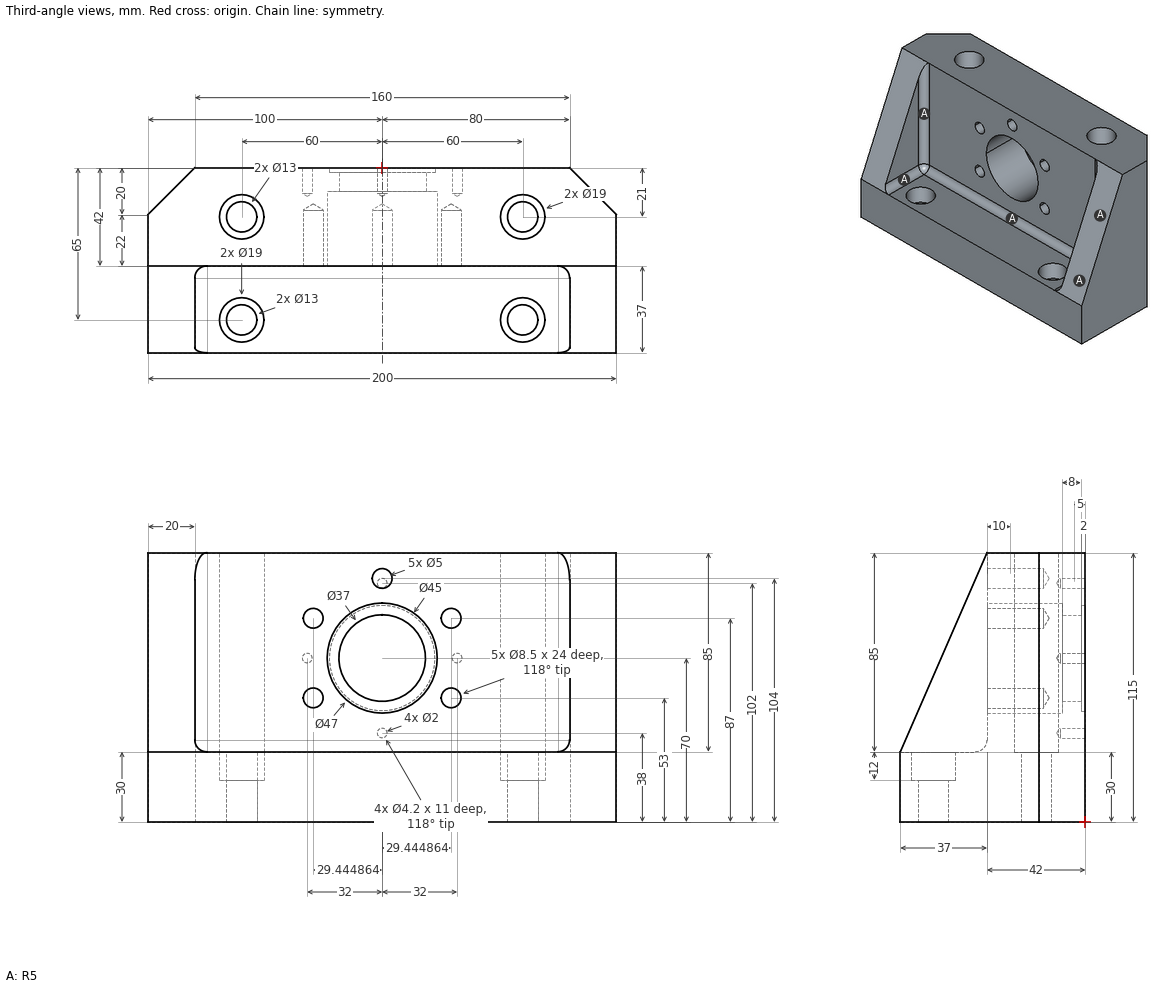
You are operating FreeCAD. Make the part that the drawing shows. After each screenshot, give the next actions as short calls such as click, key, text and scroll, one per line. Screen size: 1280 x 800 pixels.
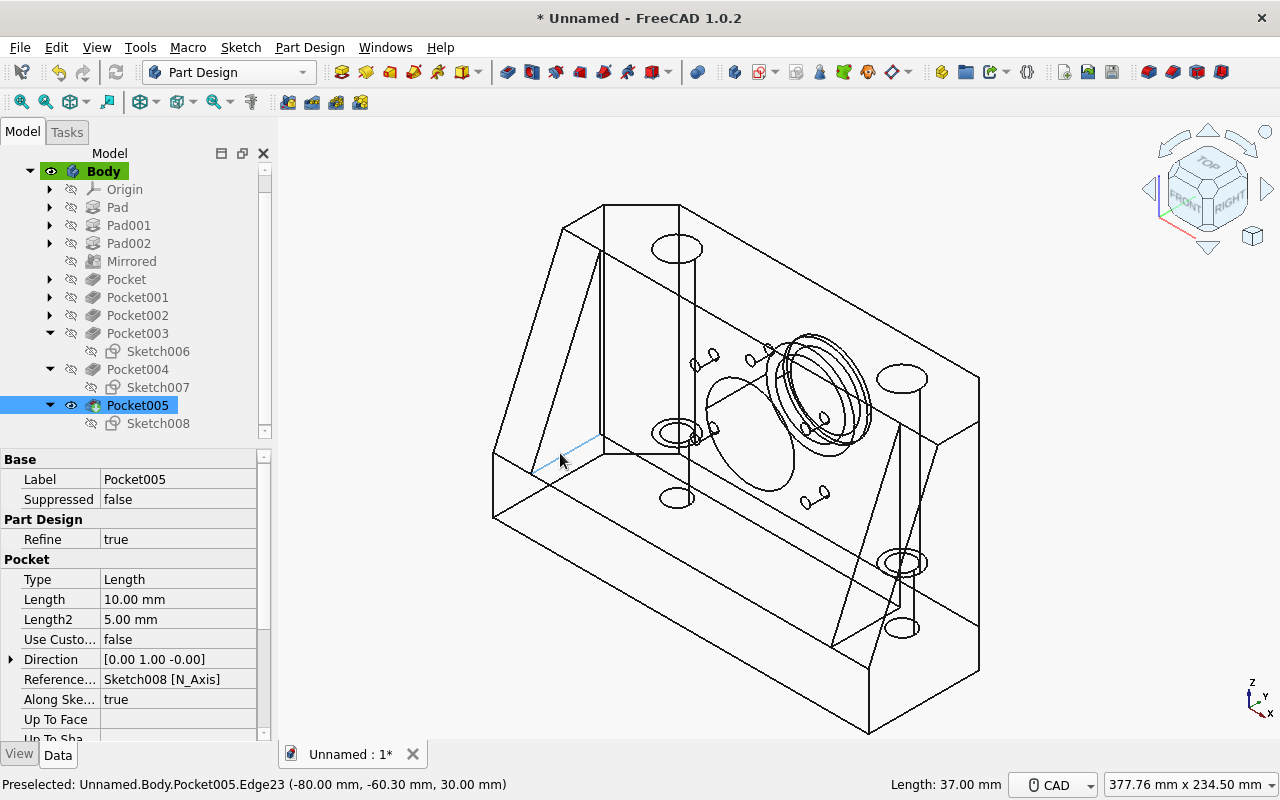
click(600, 341, ctrl)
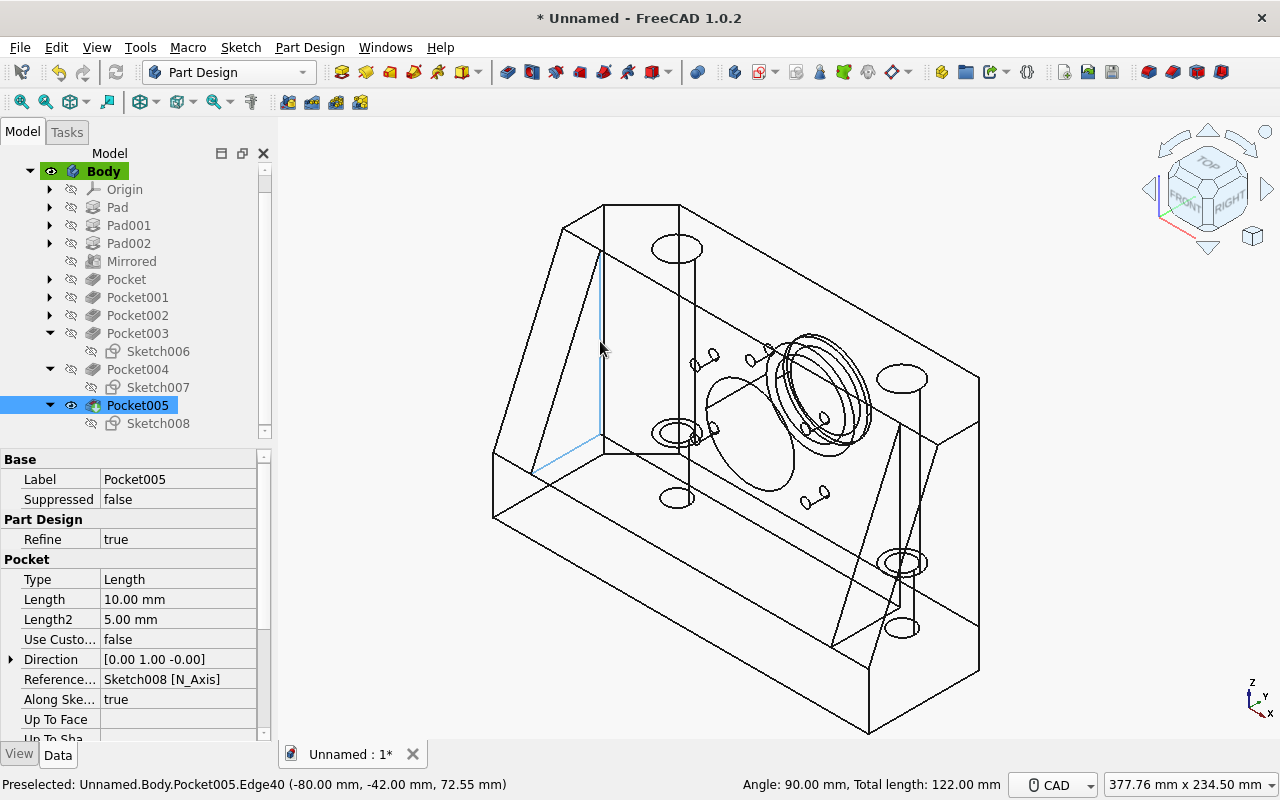
click(750, 520, ctrl)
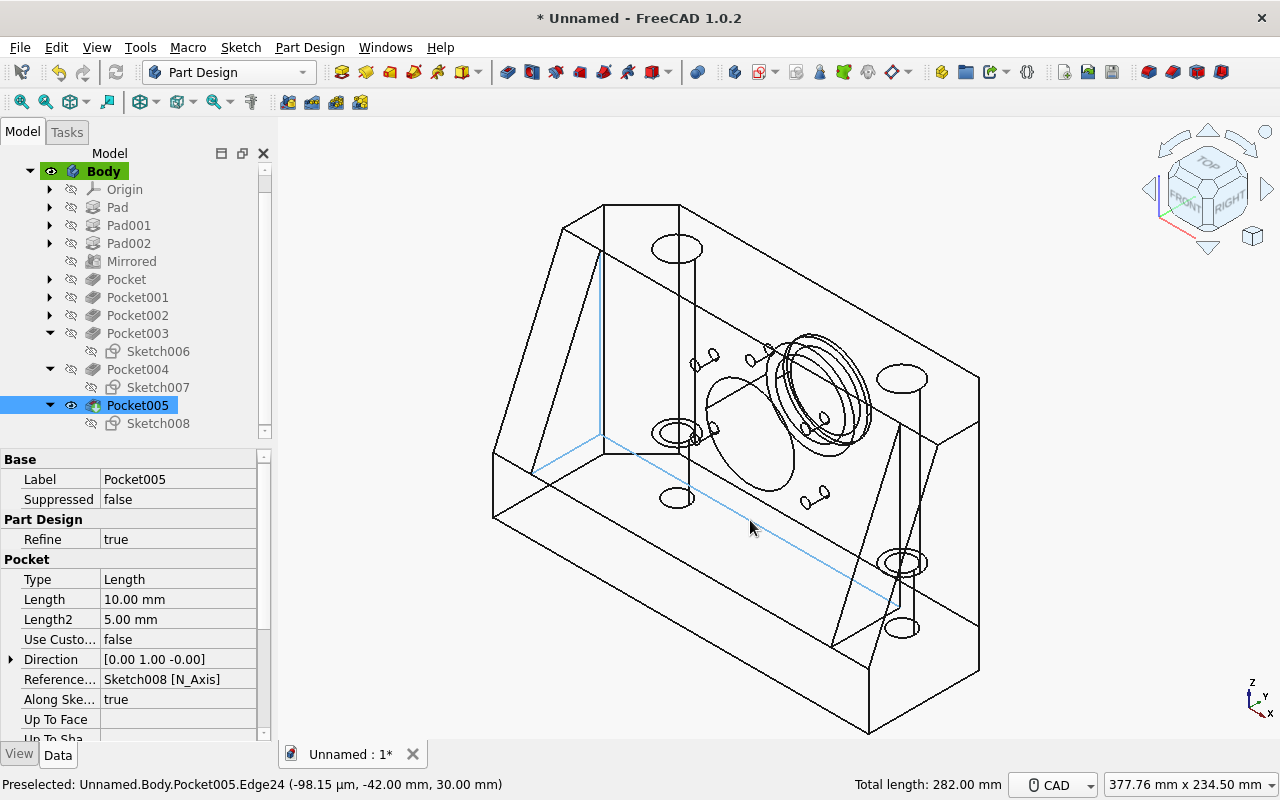
click(900, 514, ctrl)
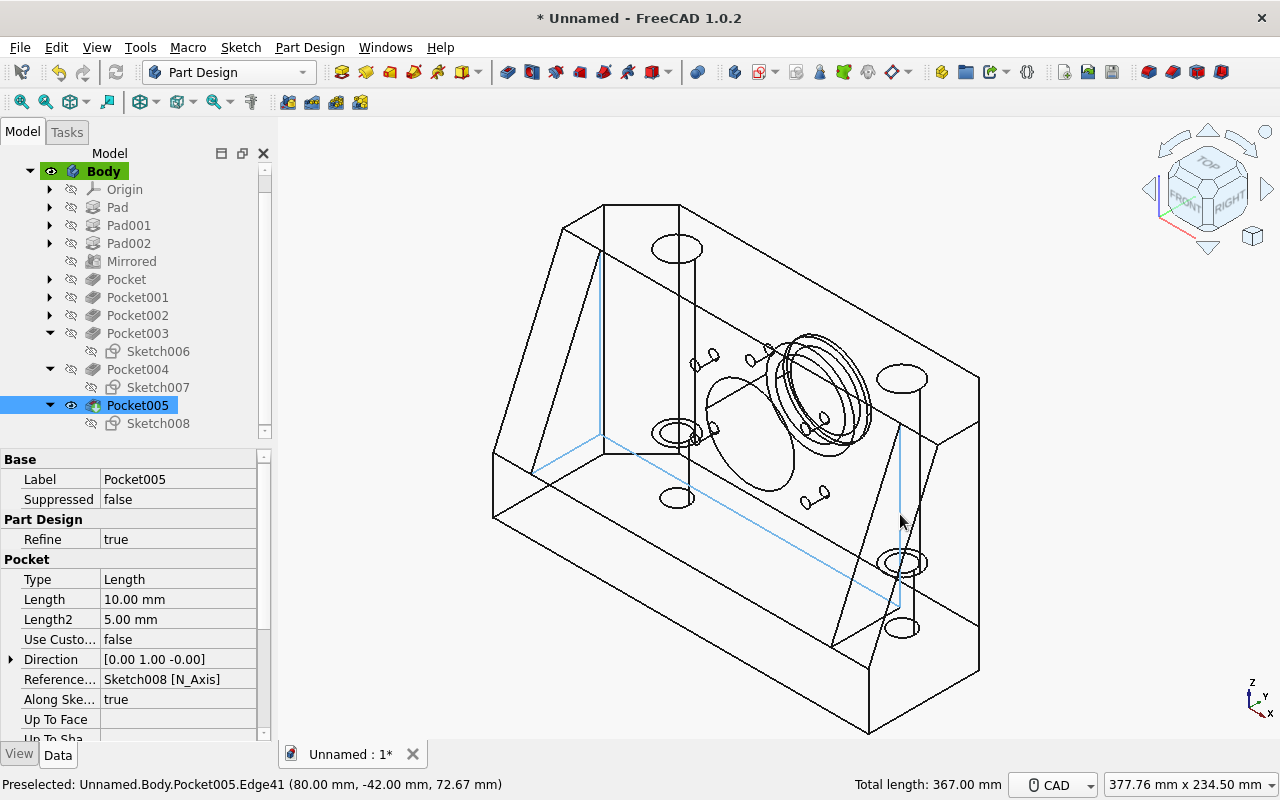
click(866, 626, ctrl)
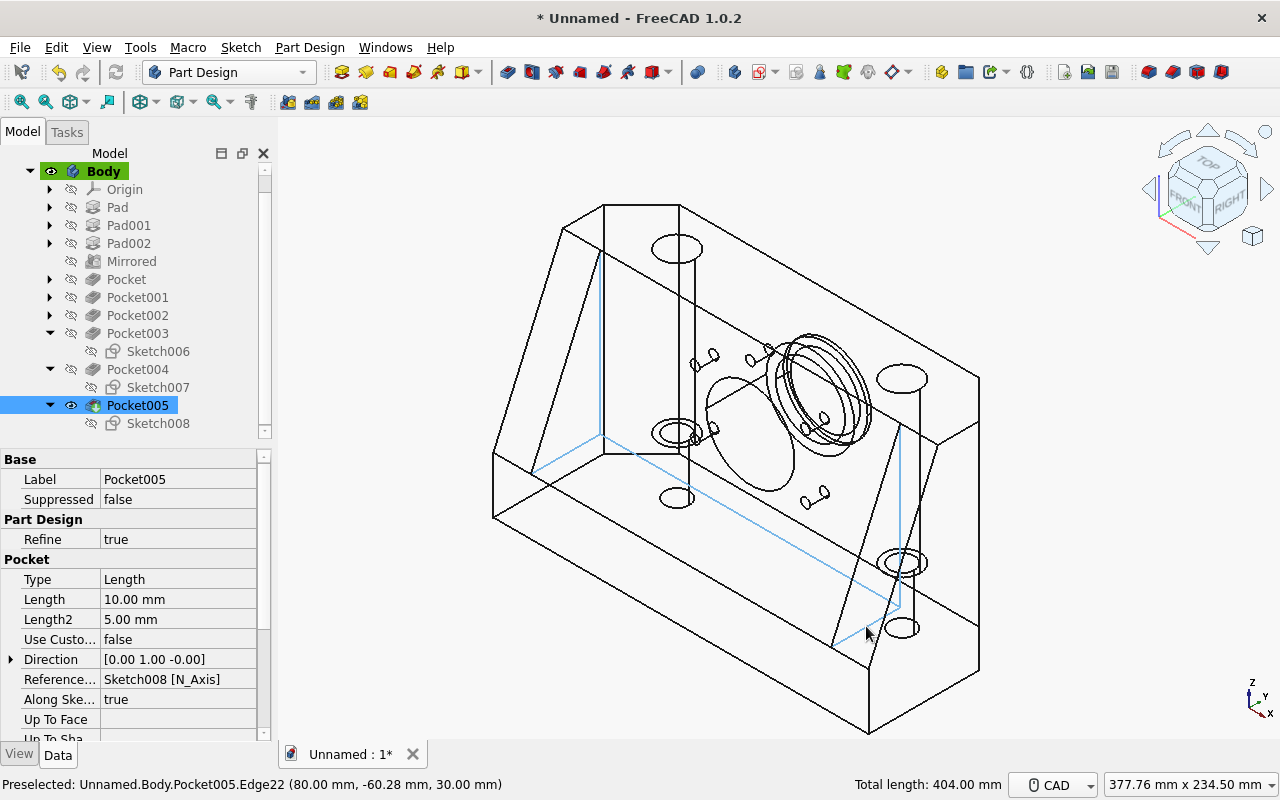
key(v)
key(1)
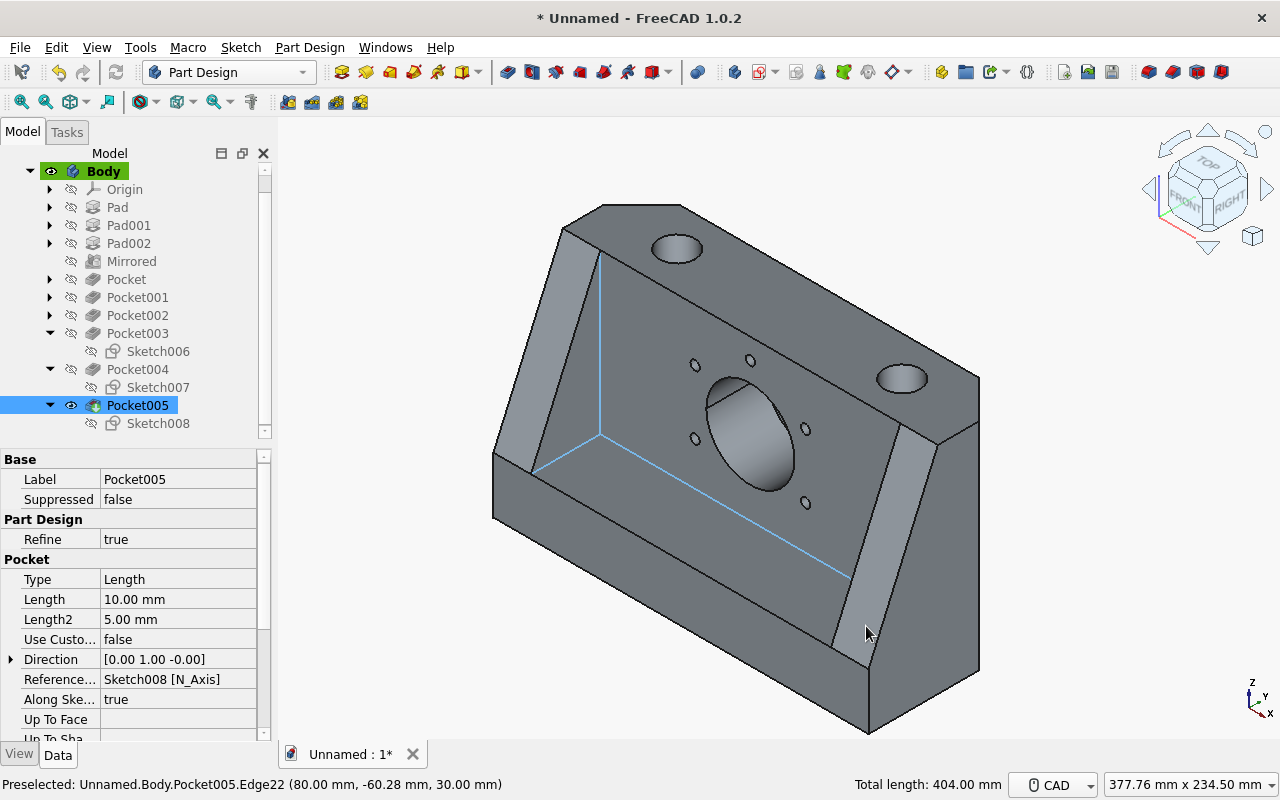
click(1150, 72)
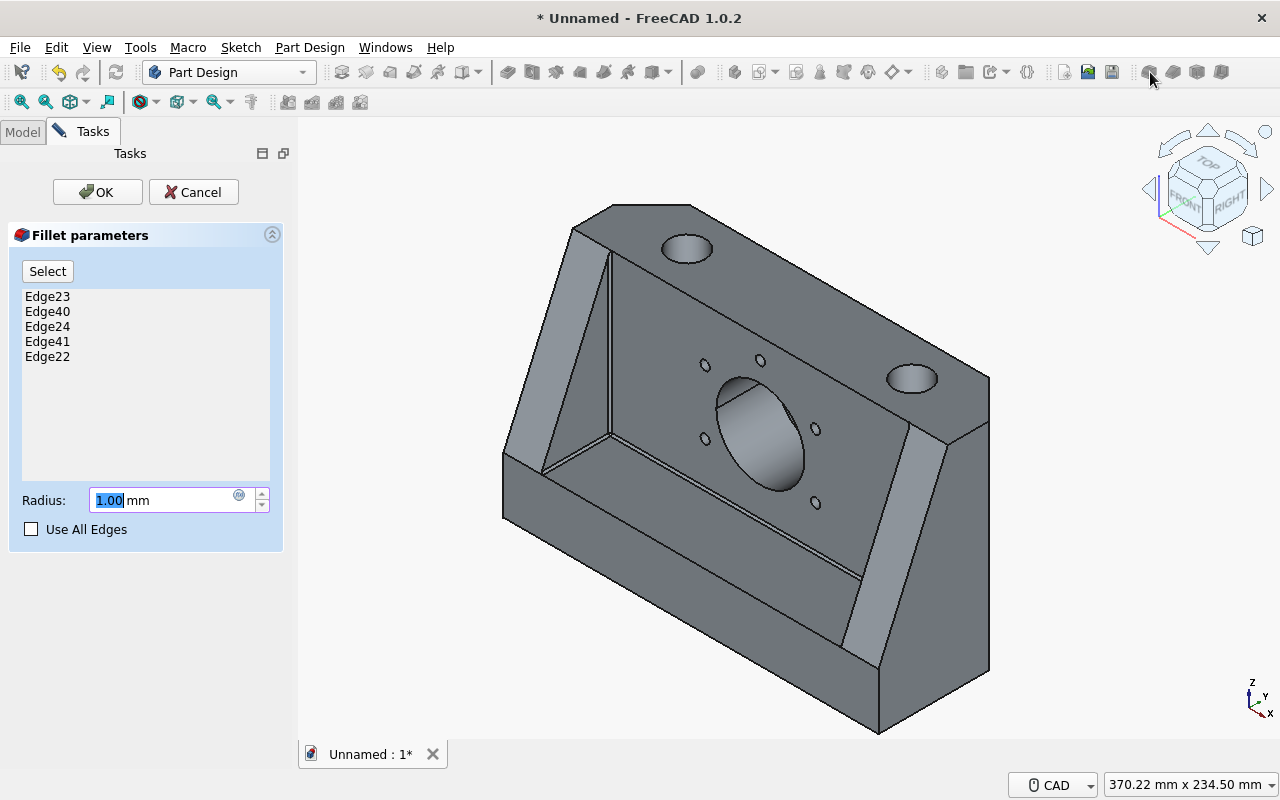
text(5)
key(Tab)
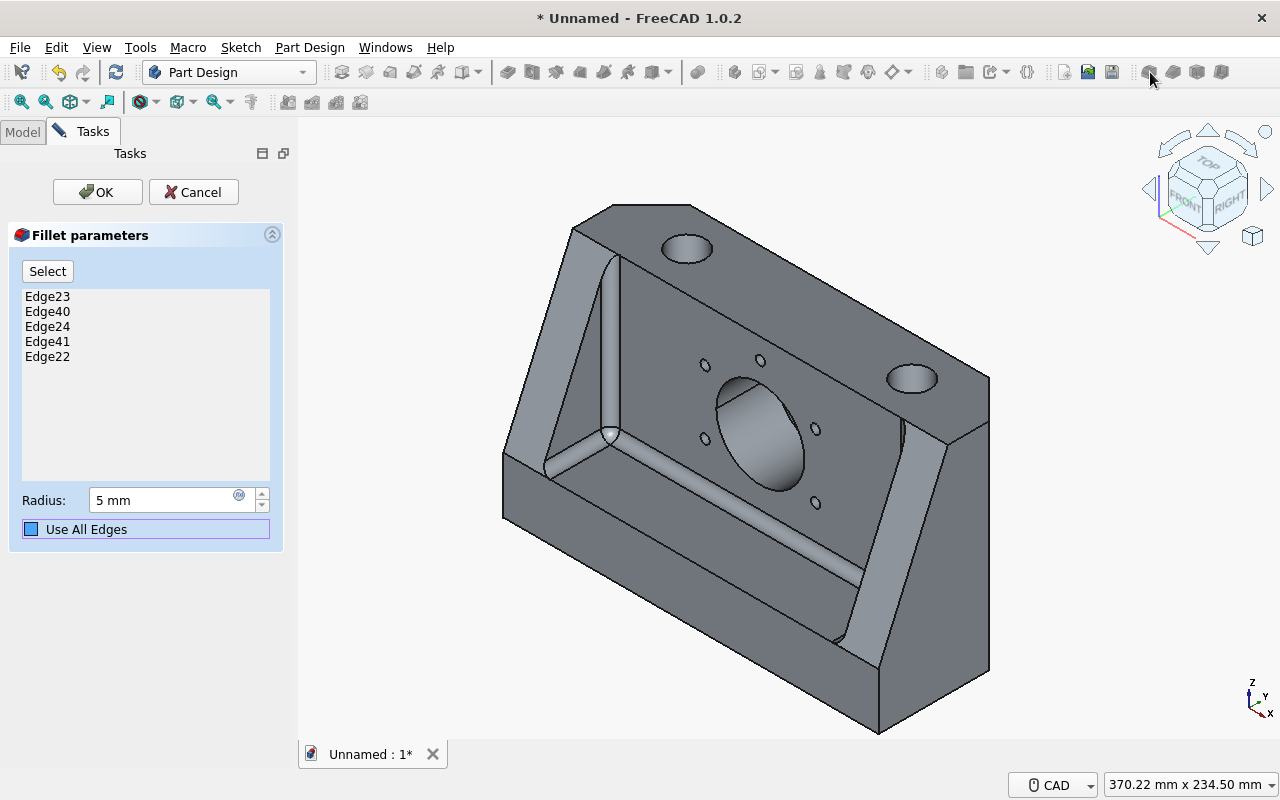
click(98, 192)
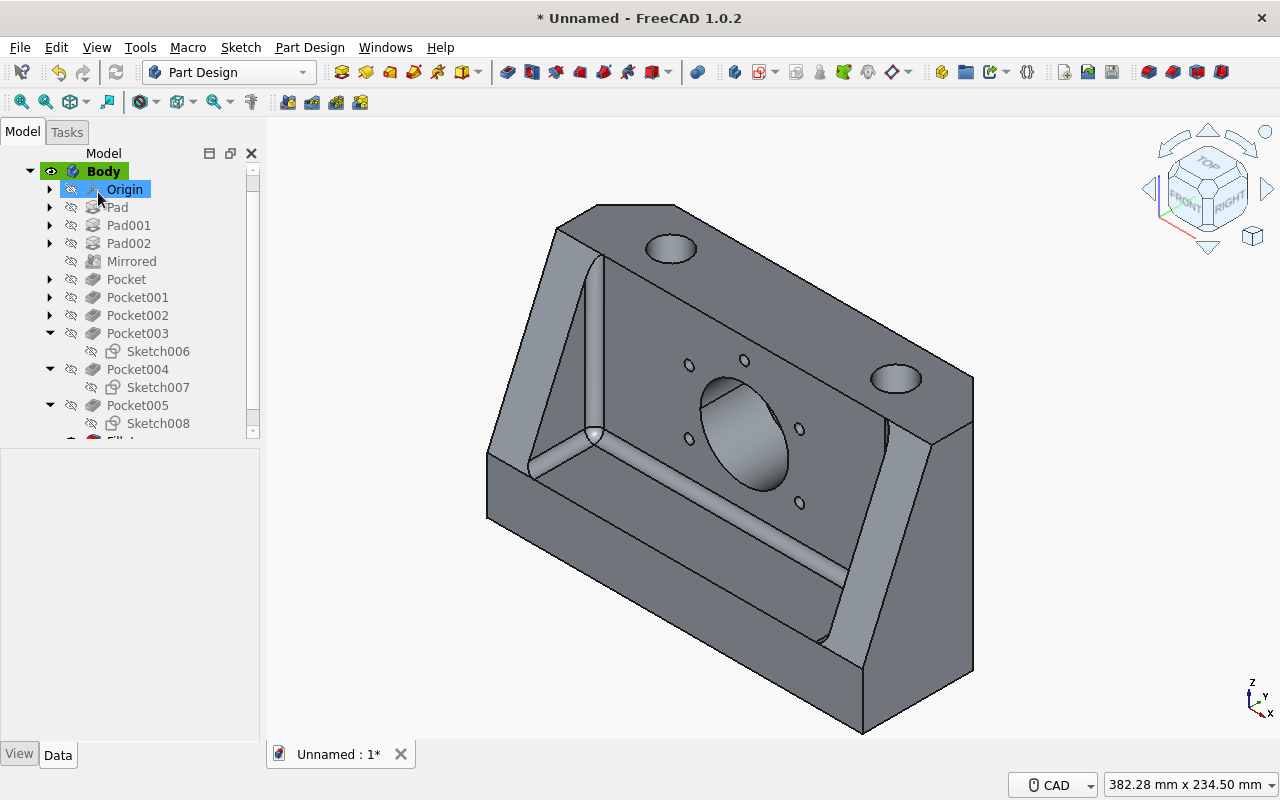
key(4)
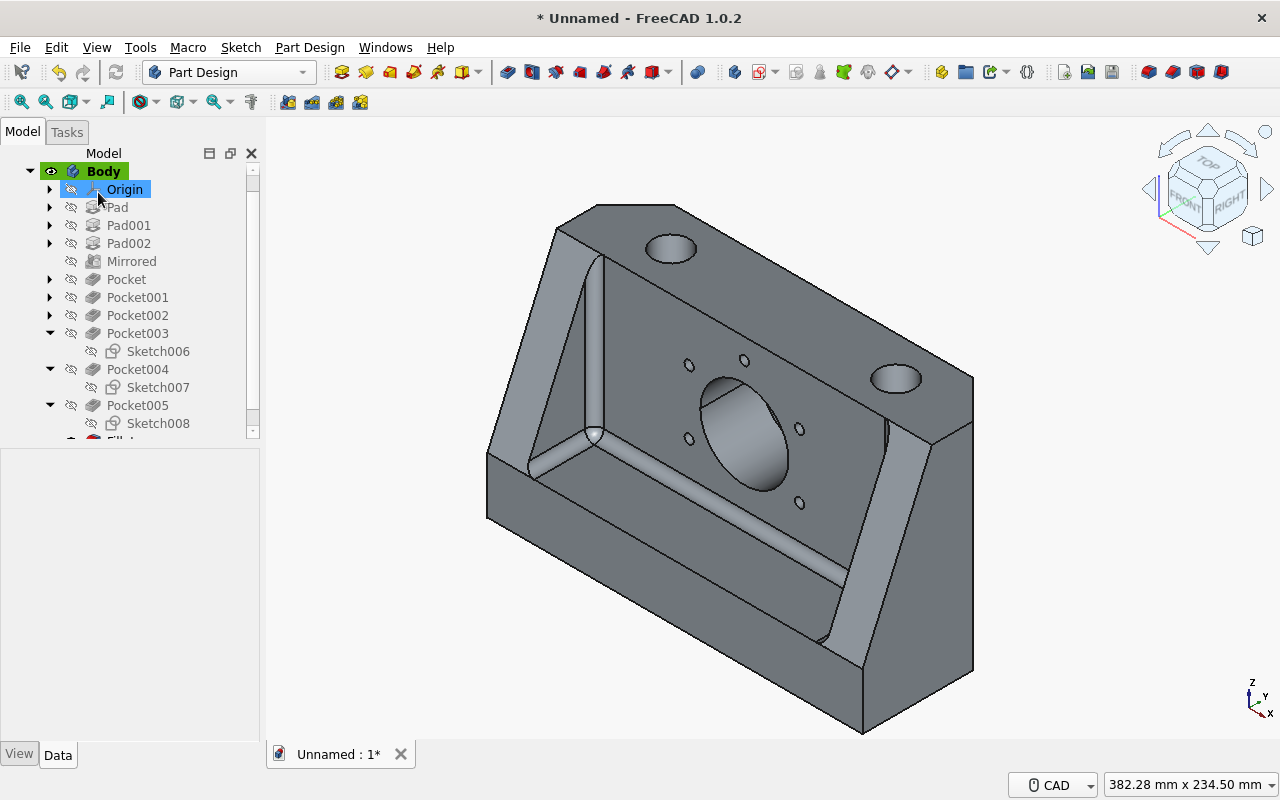
click(655, 494)